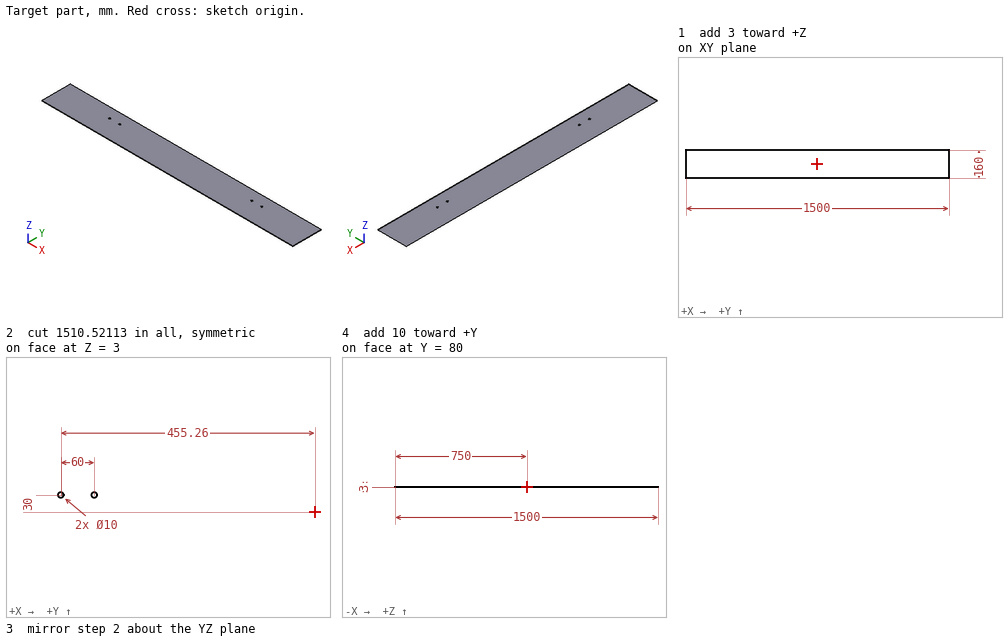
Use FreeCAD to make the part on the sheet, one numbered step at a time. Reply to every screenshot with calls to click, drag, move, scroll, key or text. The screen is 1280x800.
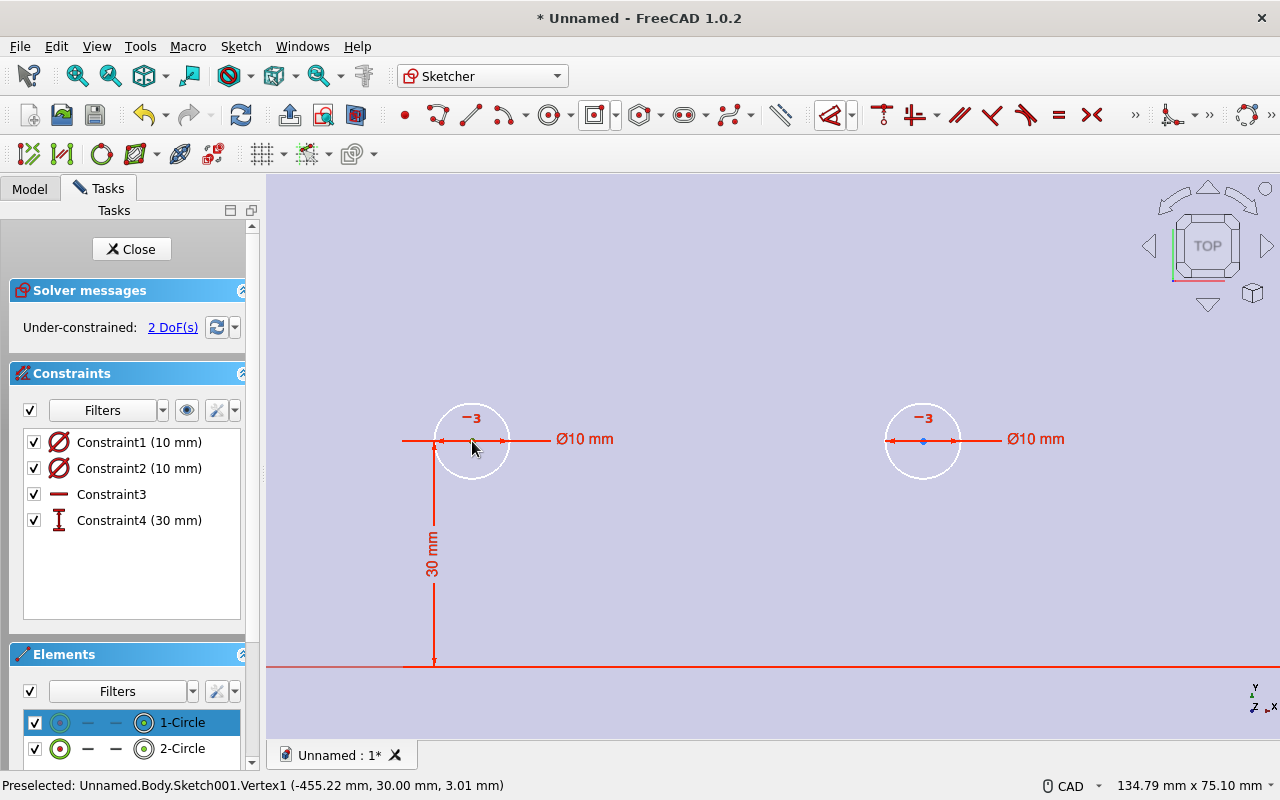
click(923, 441)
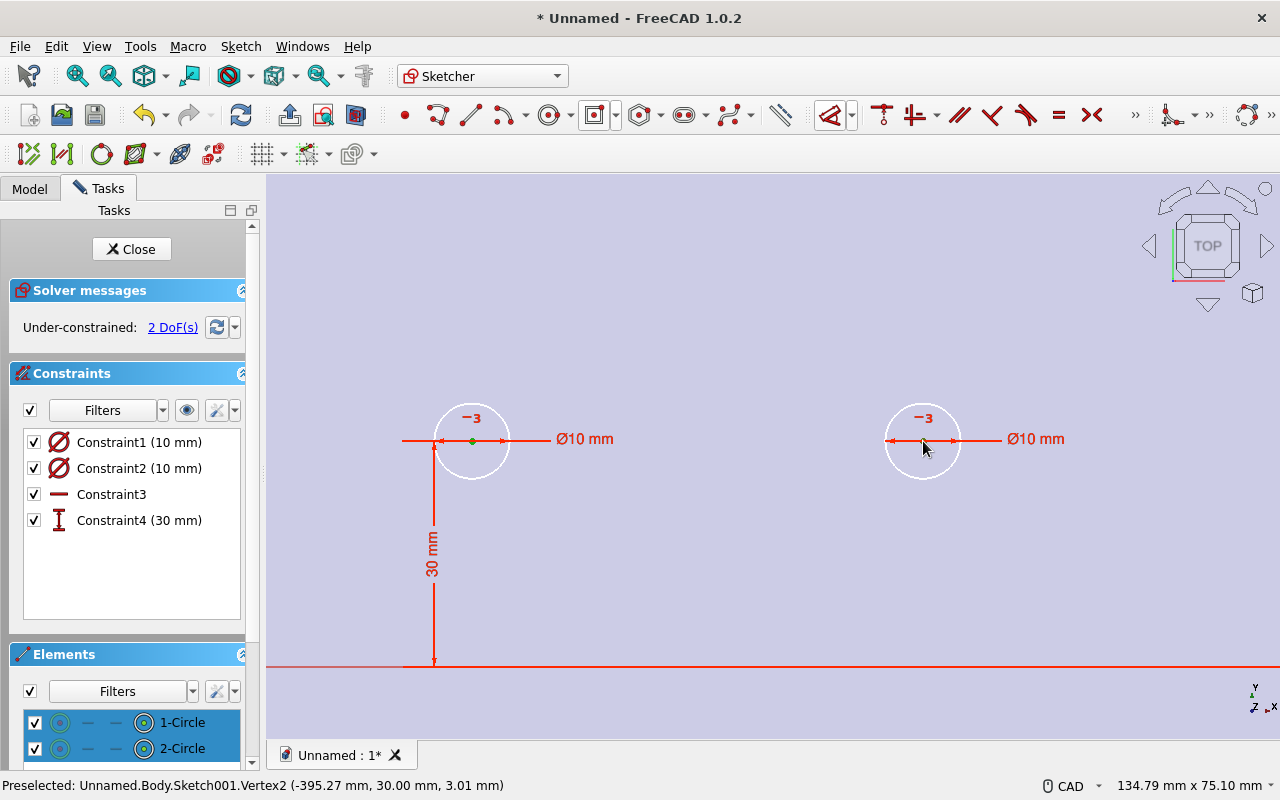
click(852, 116)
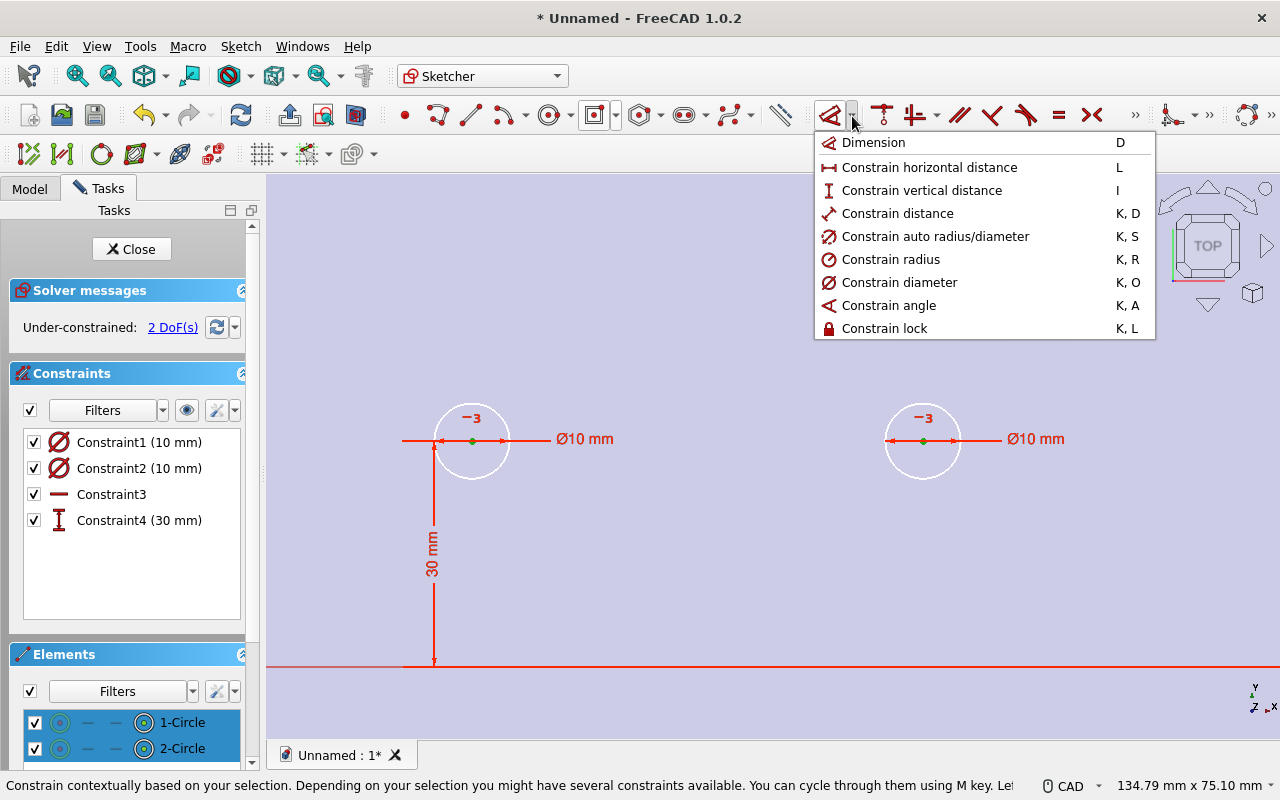
click(985, 168)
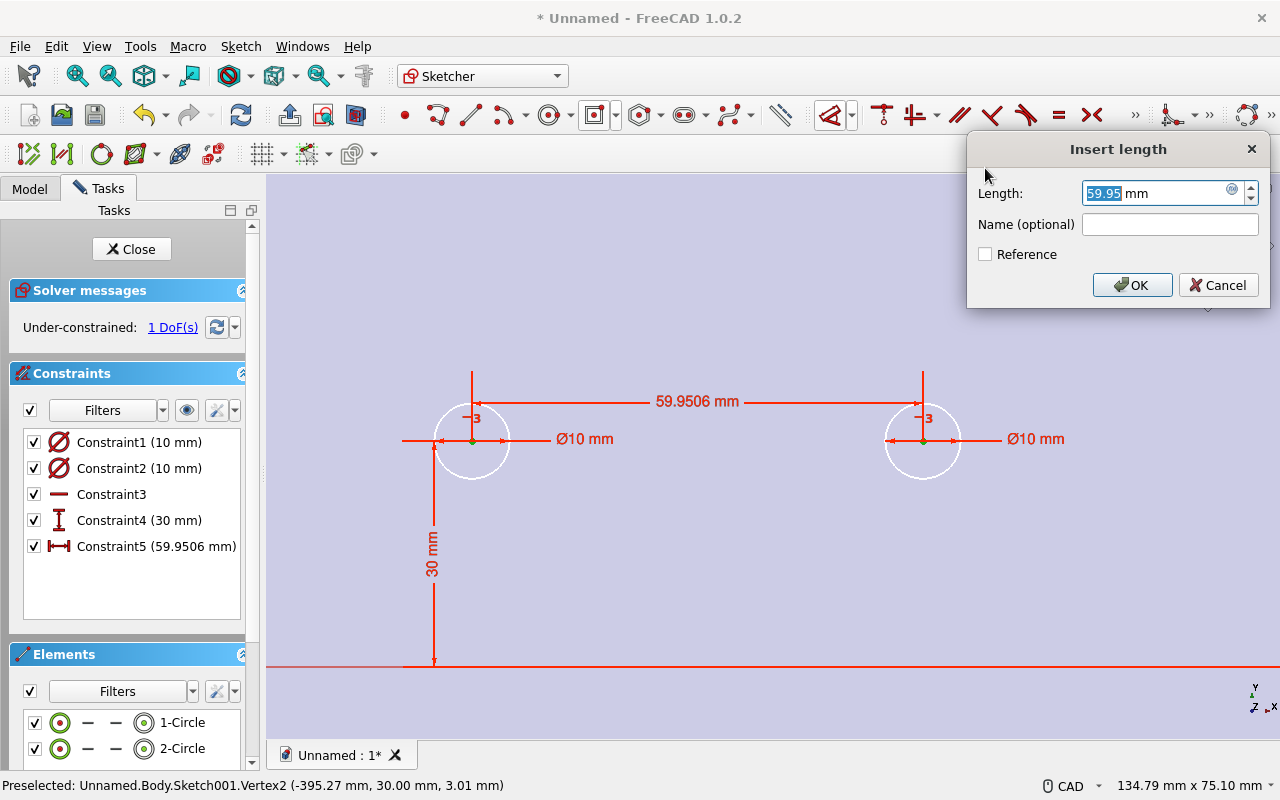
text(60)
key(Return)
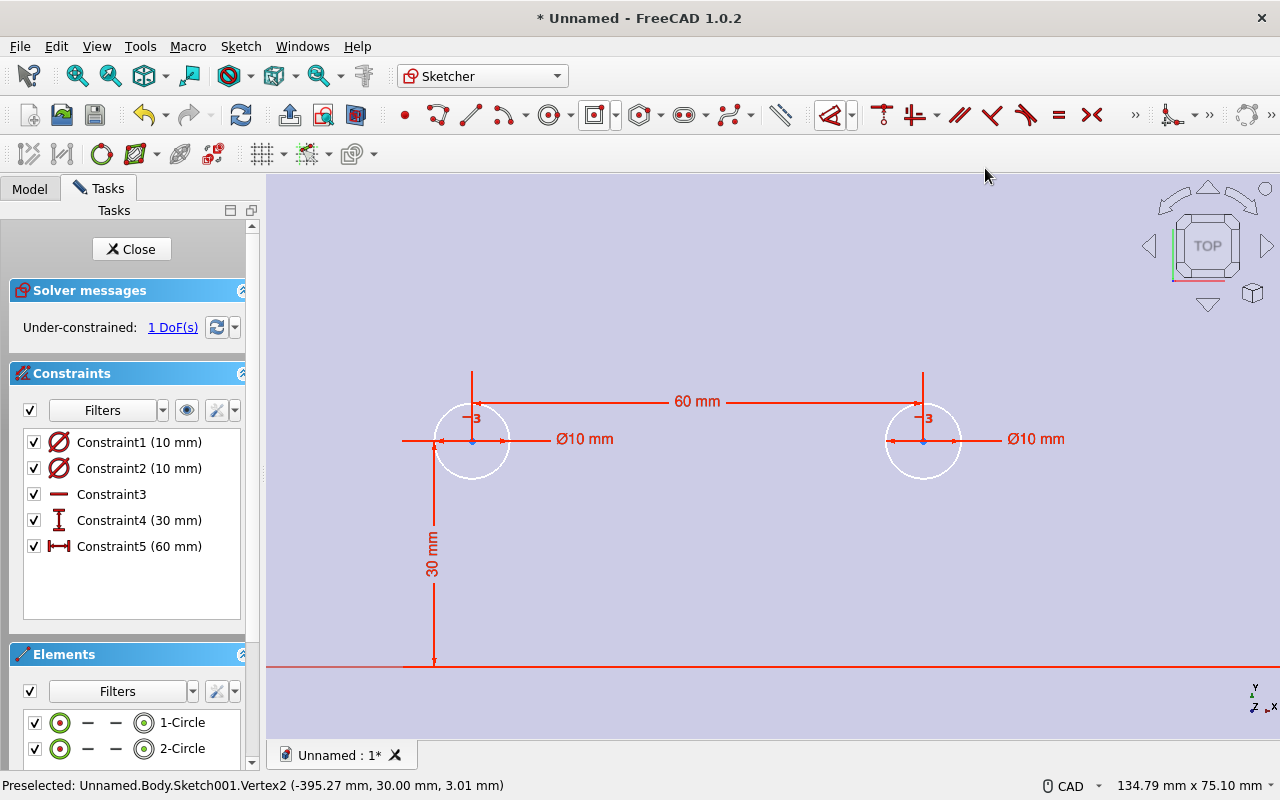
click(472, 441)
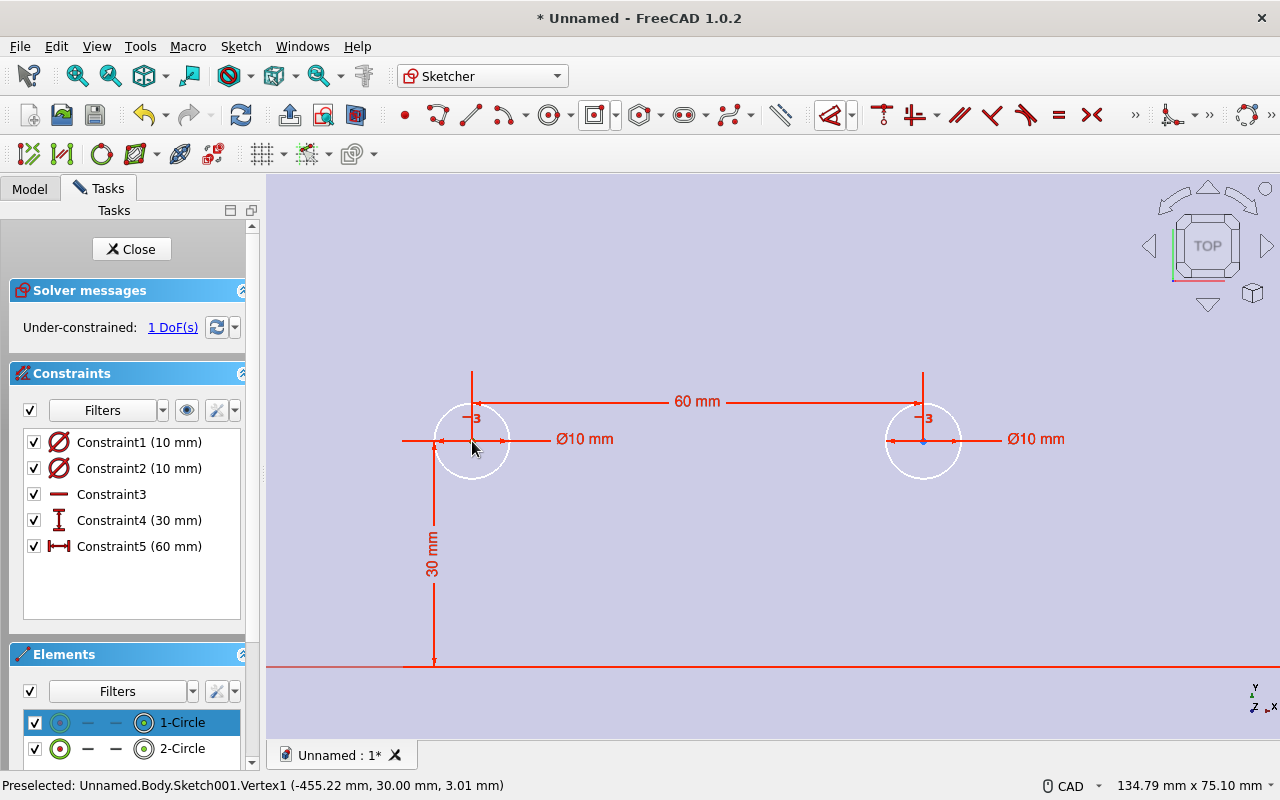
click(852, 116)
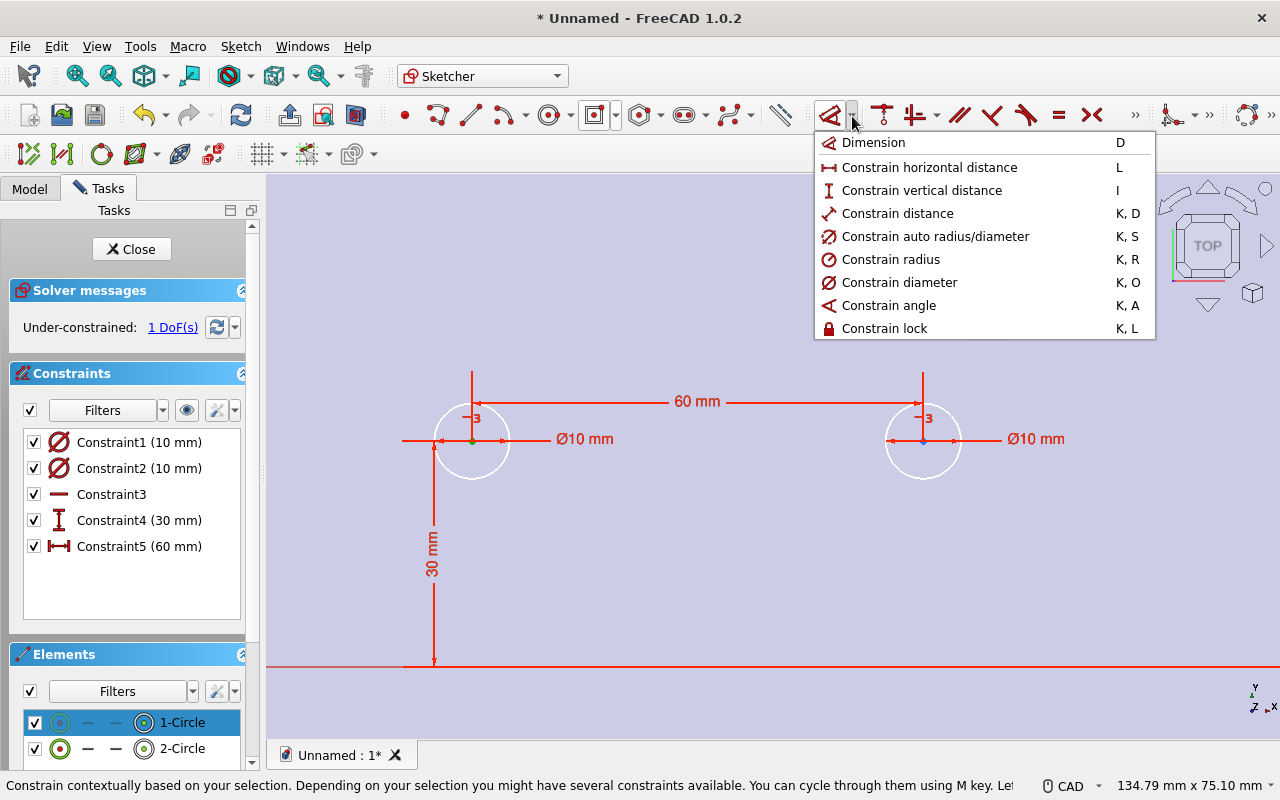
click(985, 168)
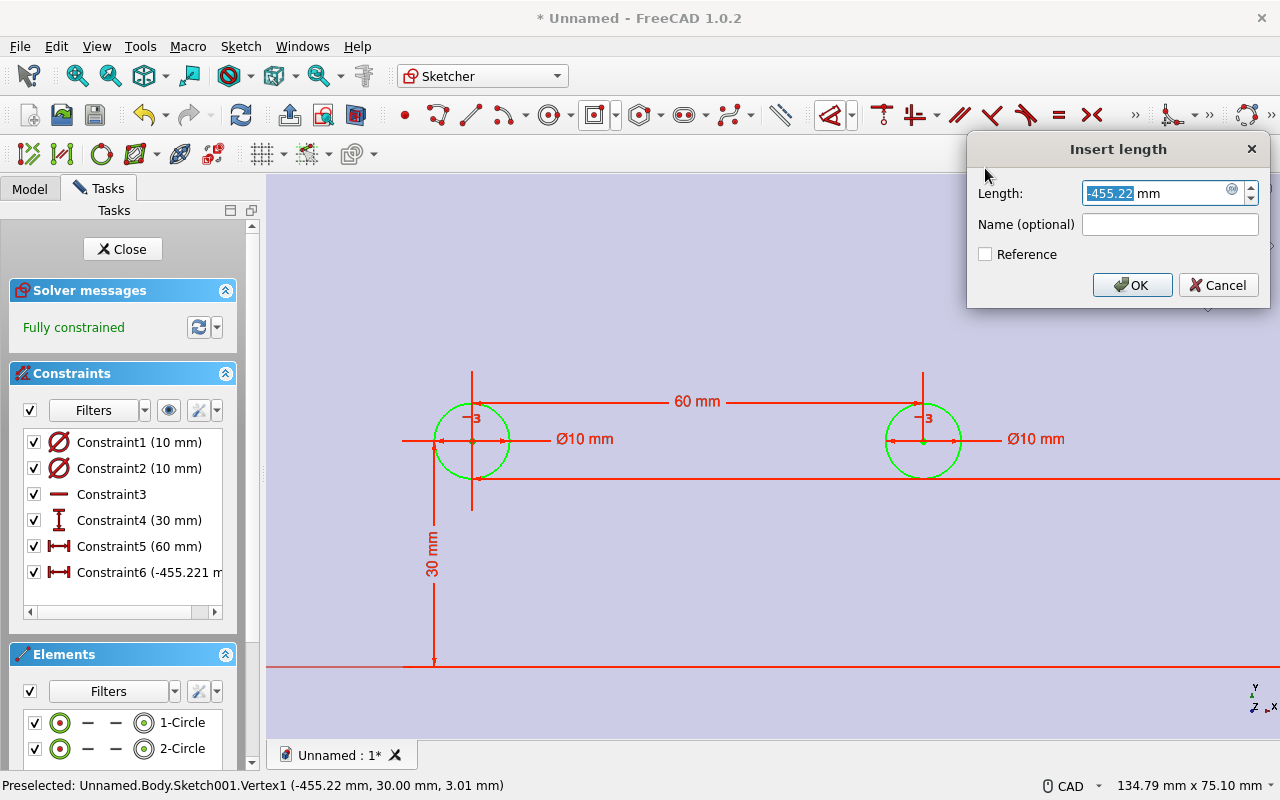
text(-455.26)
key(Return)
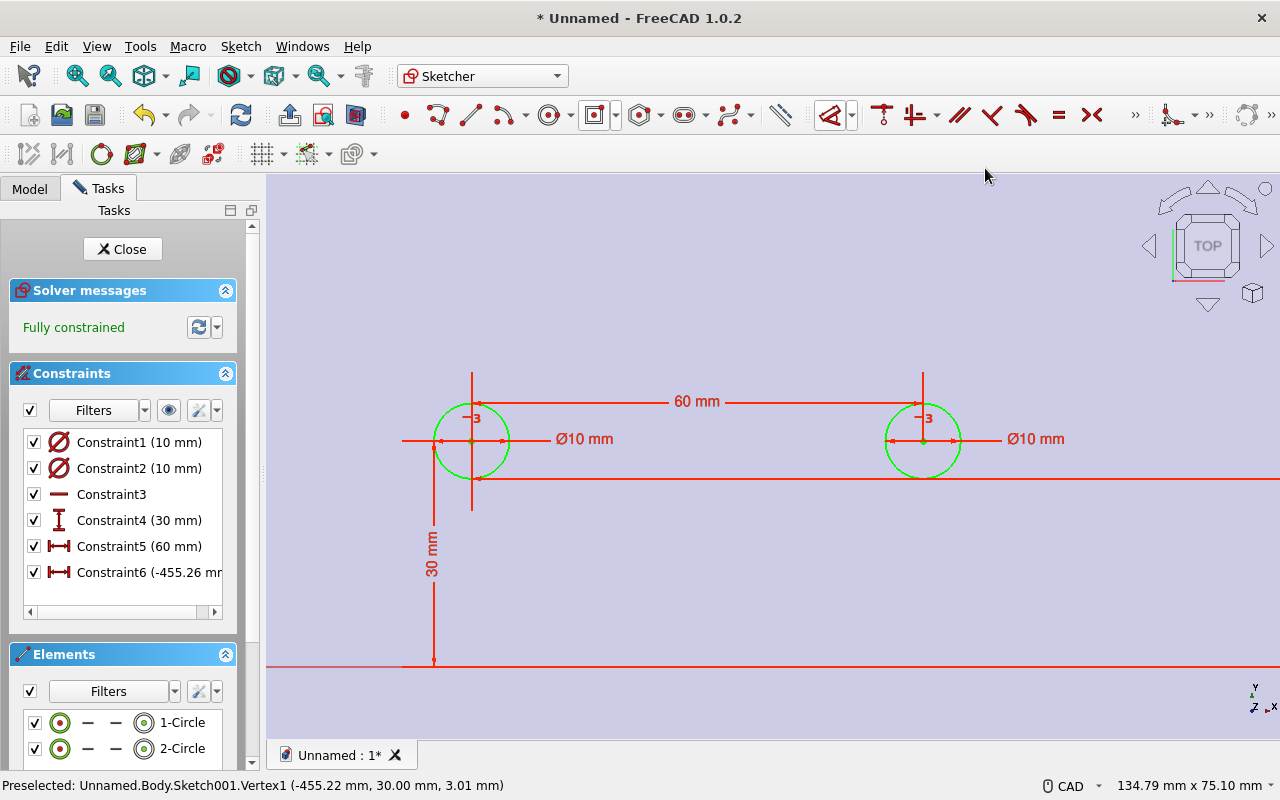
click(123, 249)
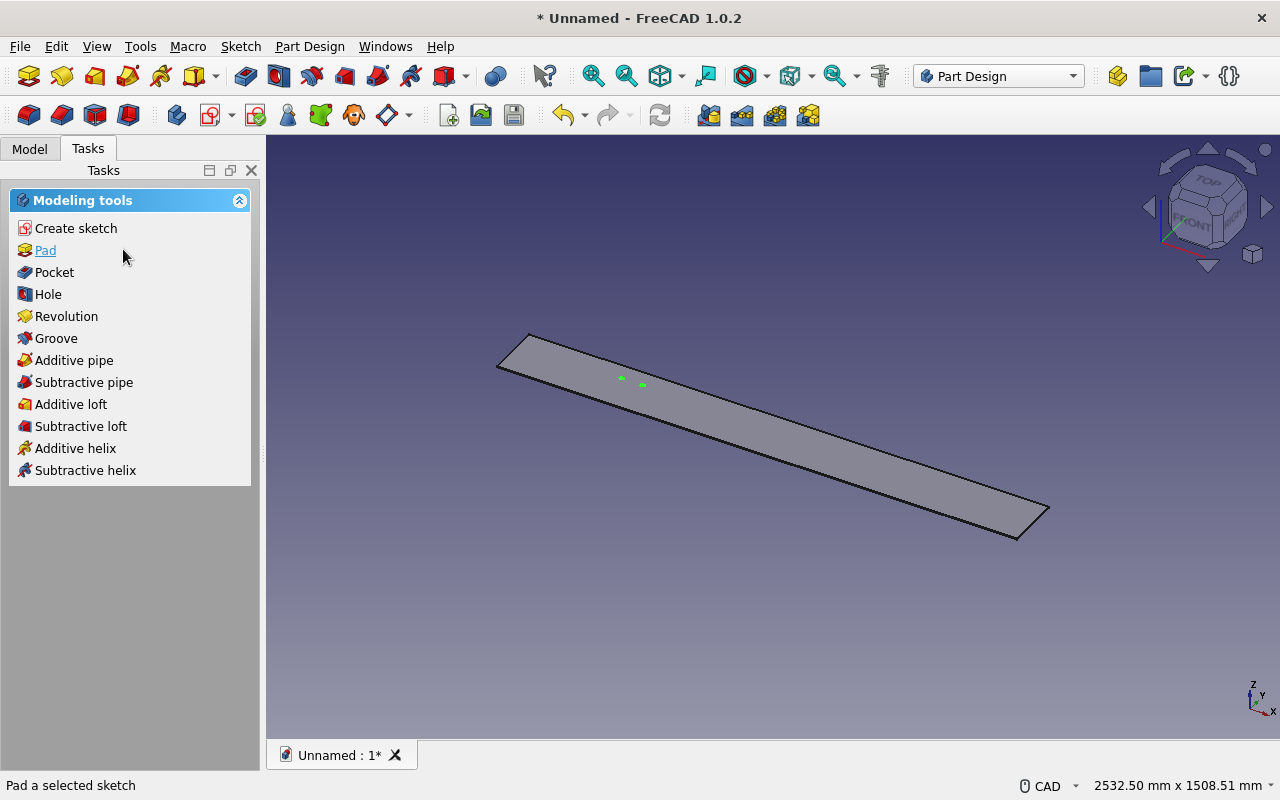
click(246, 76)